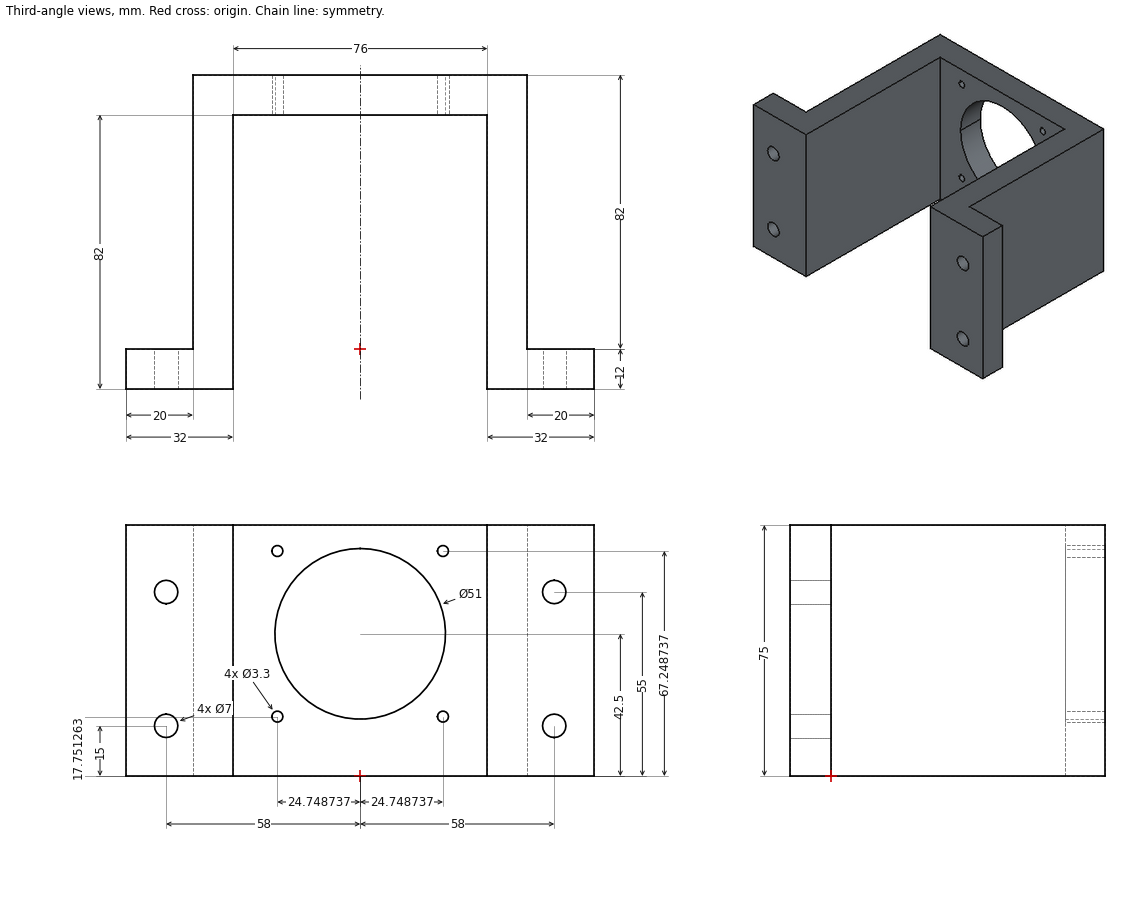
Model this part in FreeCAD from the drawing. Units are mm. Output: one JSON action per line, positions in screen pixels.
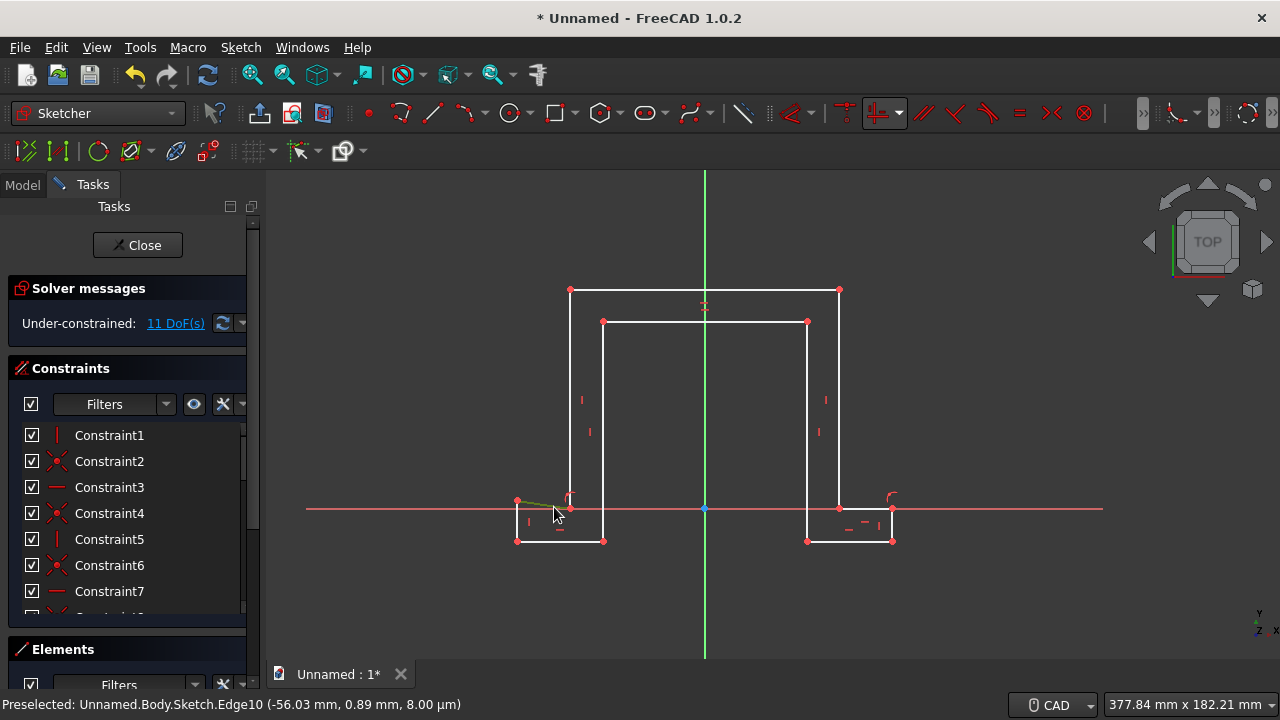
{"action": "key", "text": "h"}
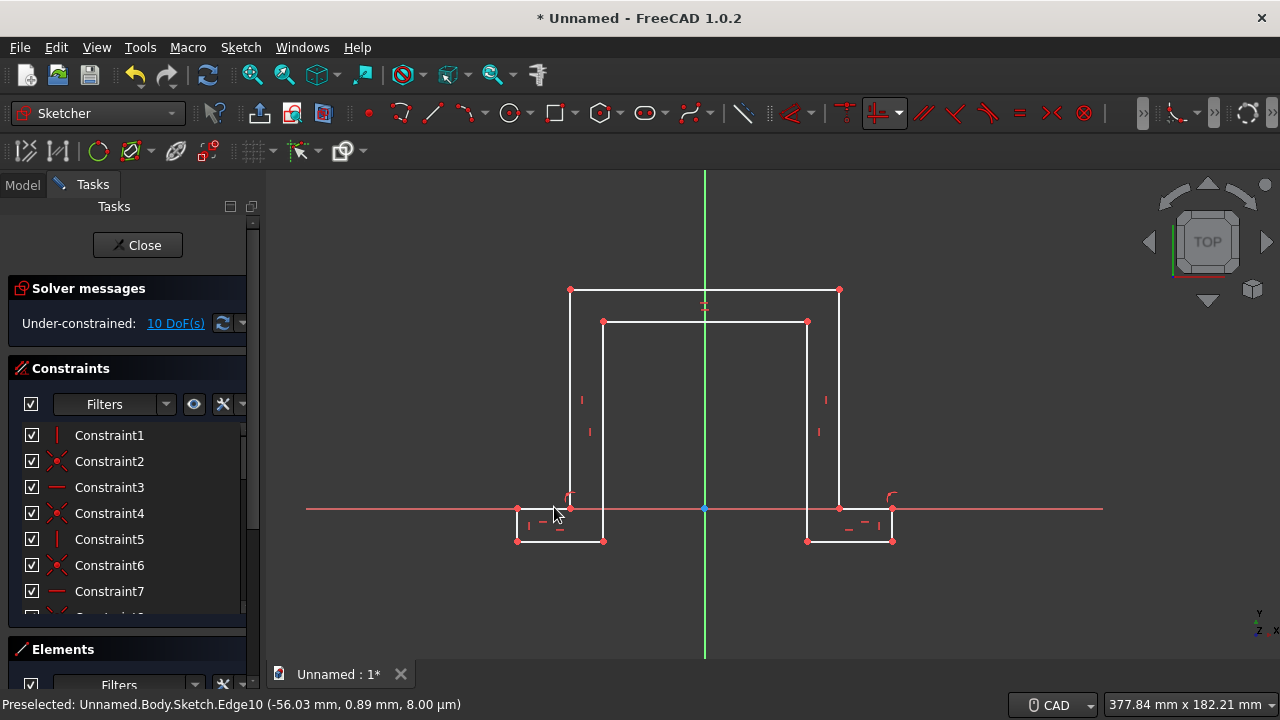
{"action": "left_click", "coordinate": [603, 542]}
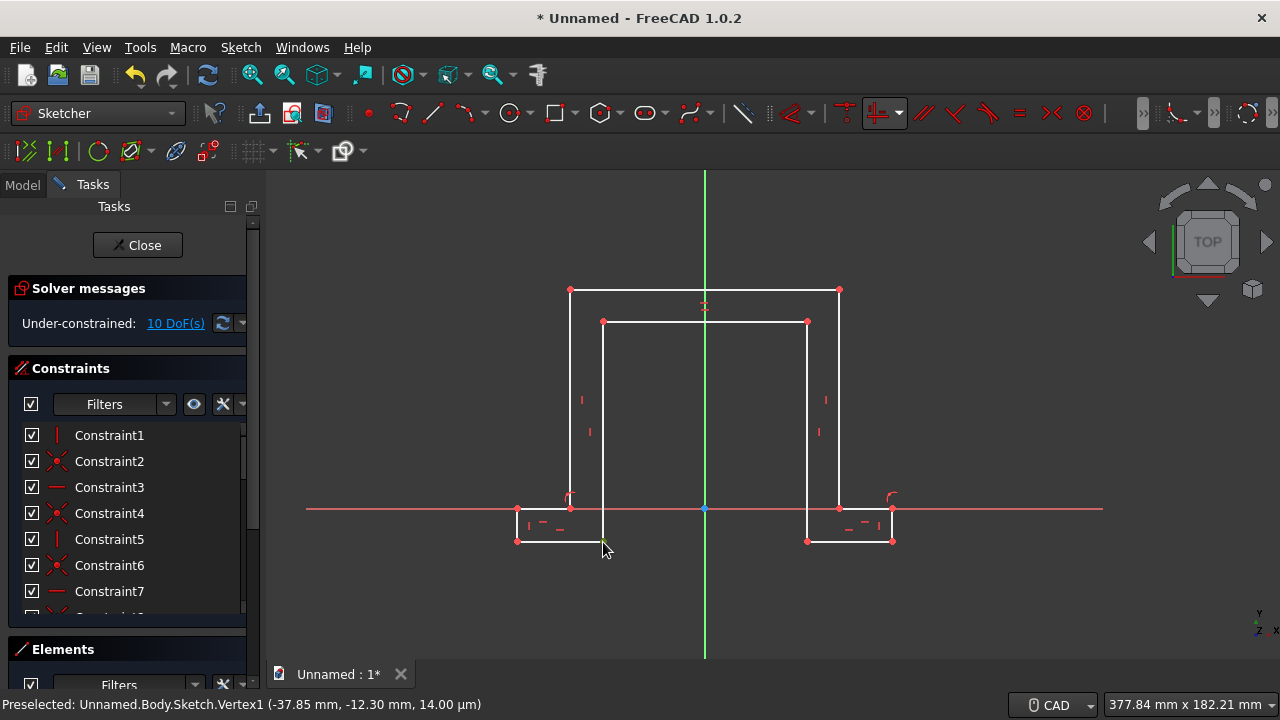
{"action": "left_click", "coordinate": [807, 542]}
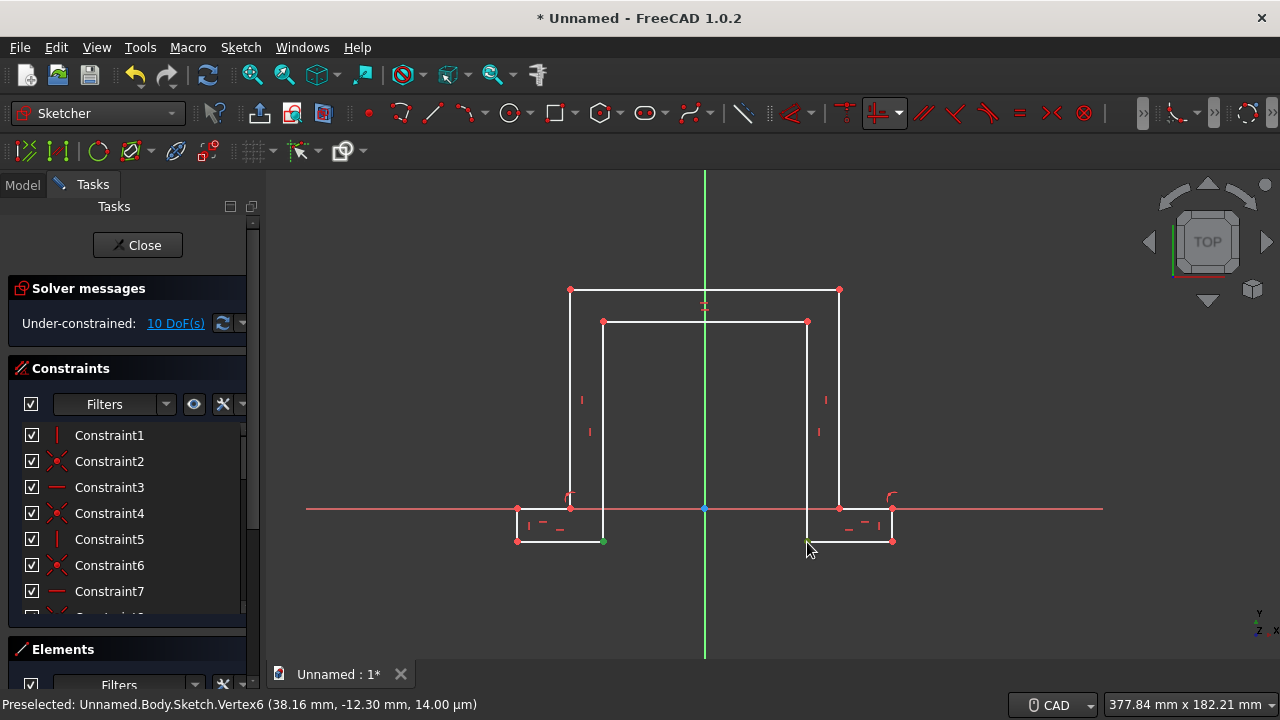
{"action": "left_click", "coordinate": [705, 600]}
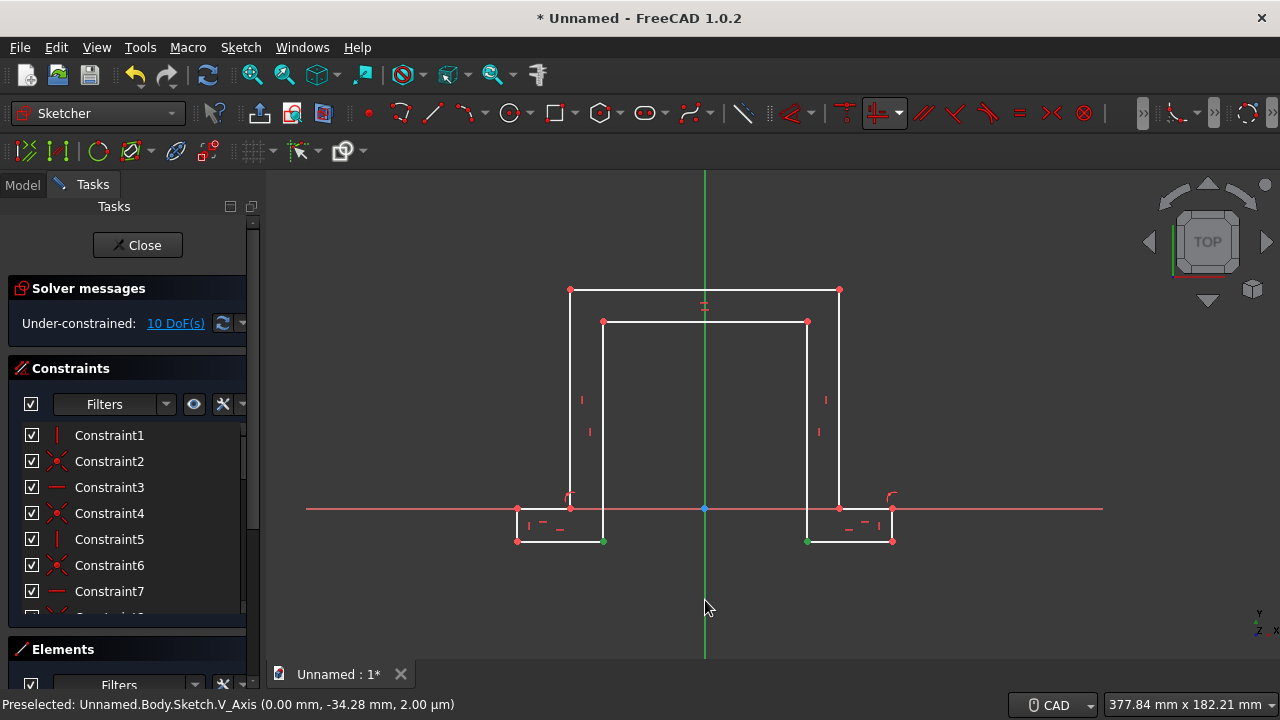
{"action": "left_click", "coordinate": [1052, 114]}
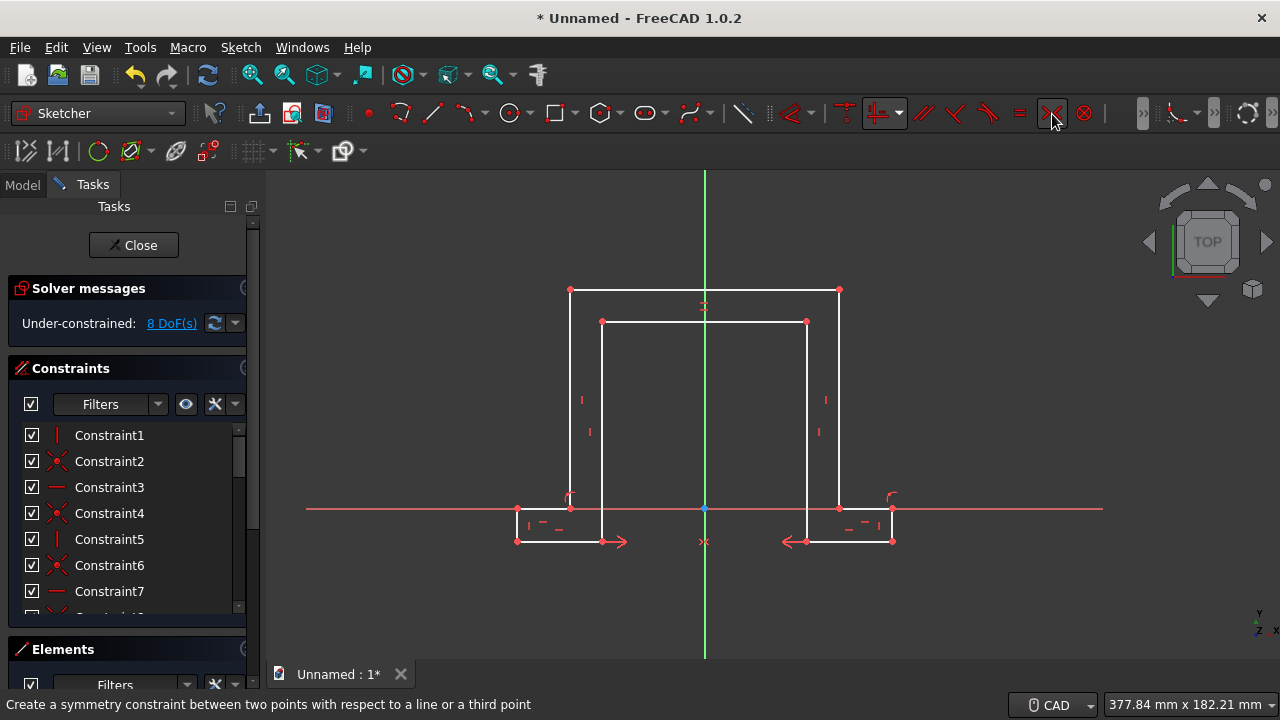
{"action": "left_click", "coordinate": [790, 114]}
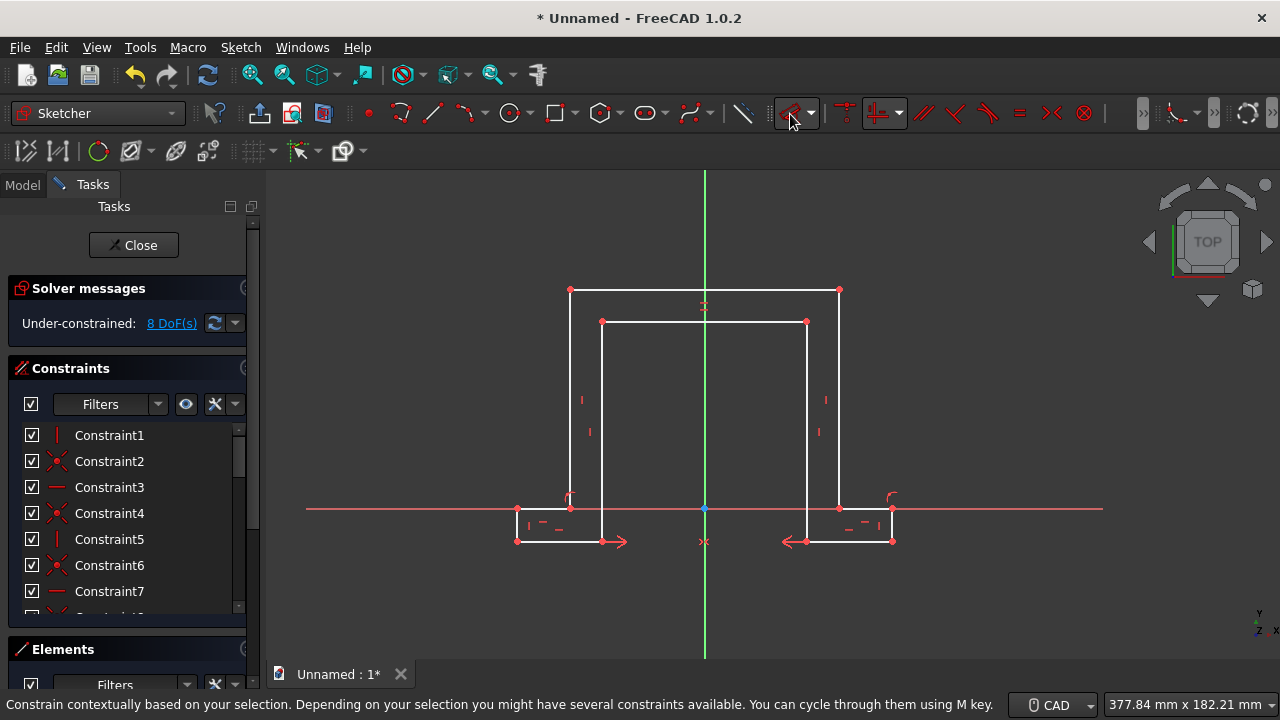
{"action": "left_click", "coordinate": [602, 476]}
{"action": "left_click", "coordinate": [636, 432]}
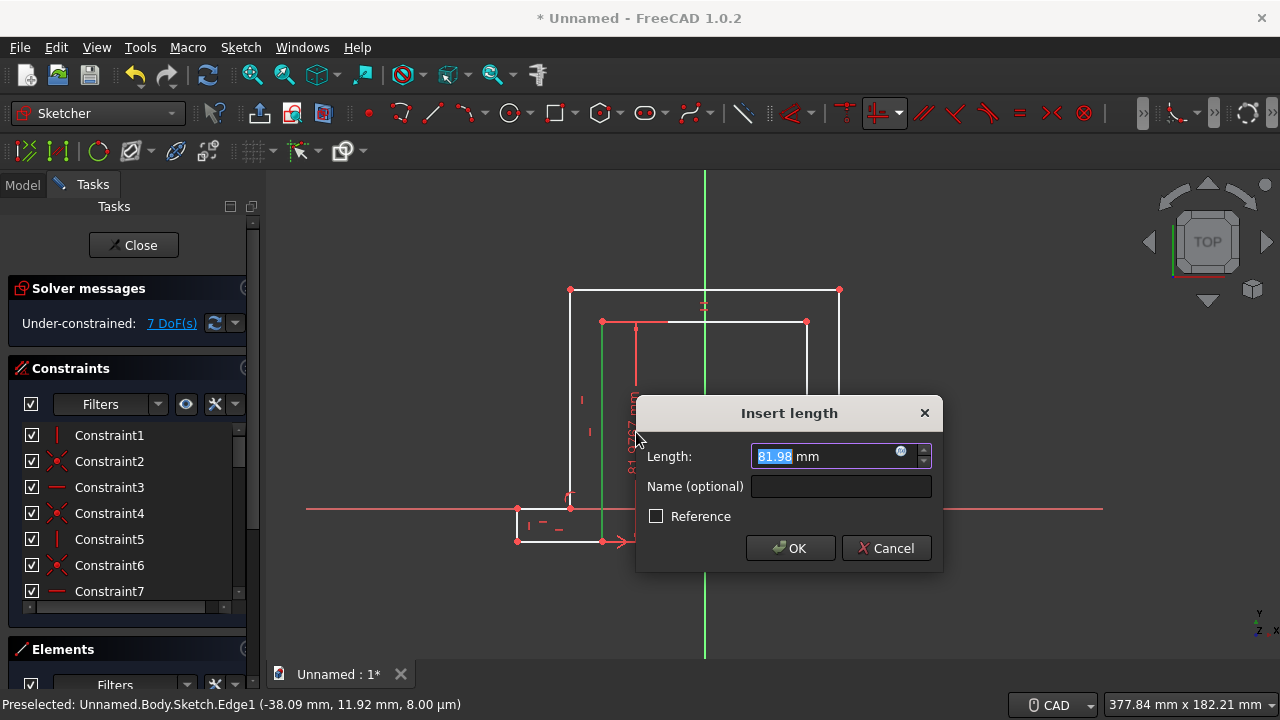
{"action": "type", "text": "82"}
{"action": "key", "text": "Return"}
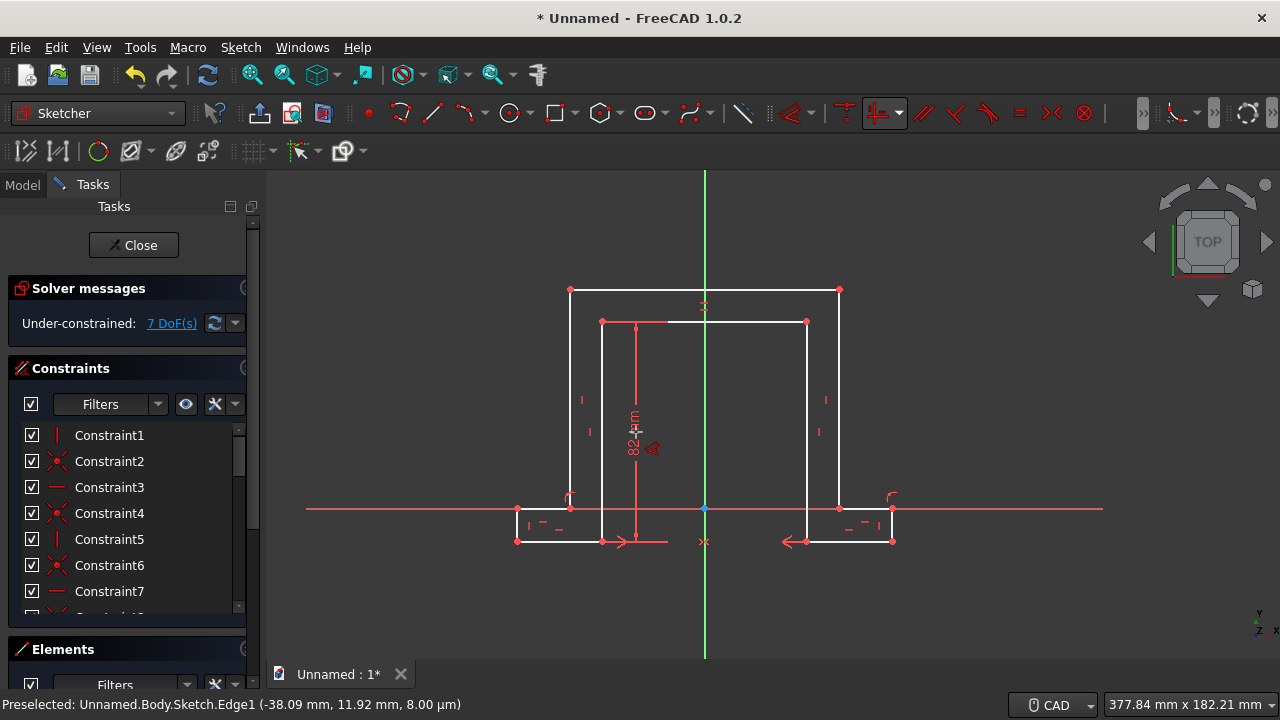
{"action": "left_click", "coordinate": [664, 322]}
{"action": "left_click", "coordinate": [658, 356]}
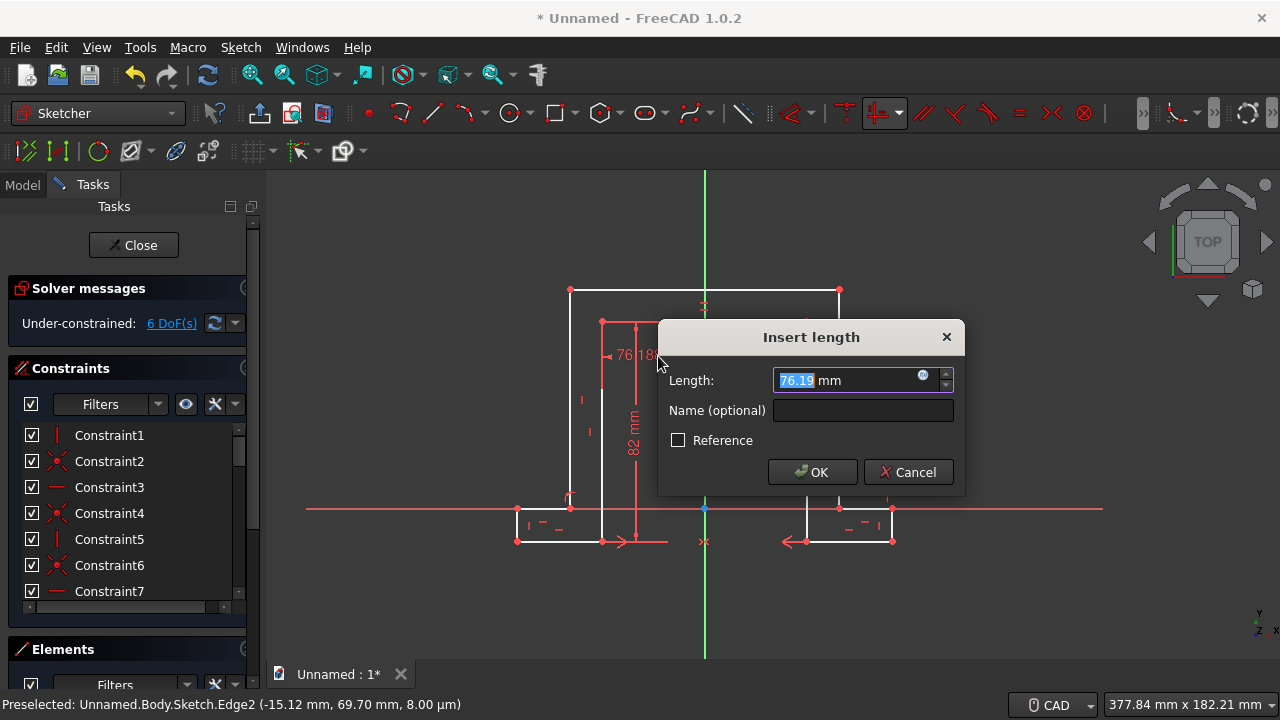
{"action": "type", "text": "76"}
{"action": "key", "text": "Return"}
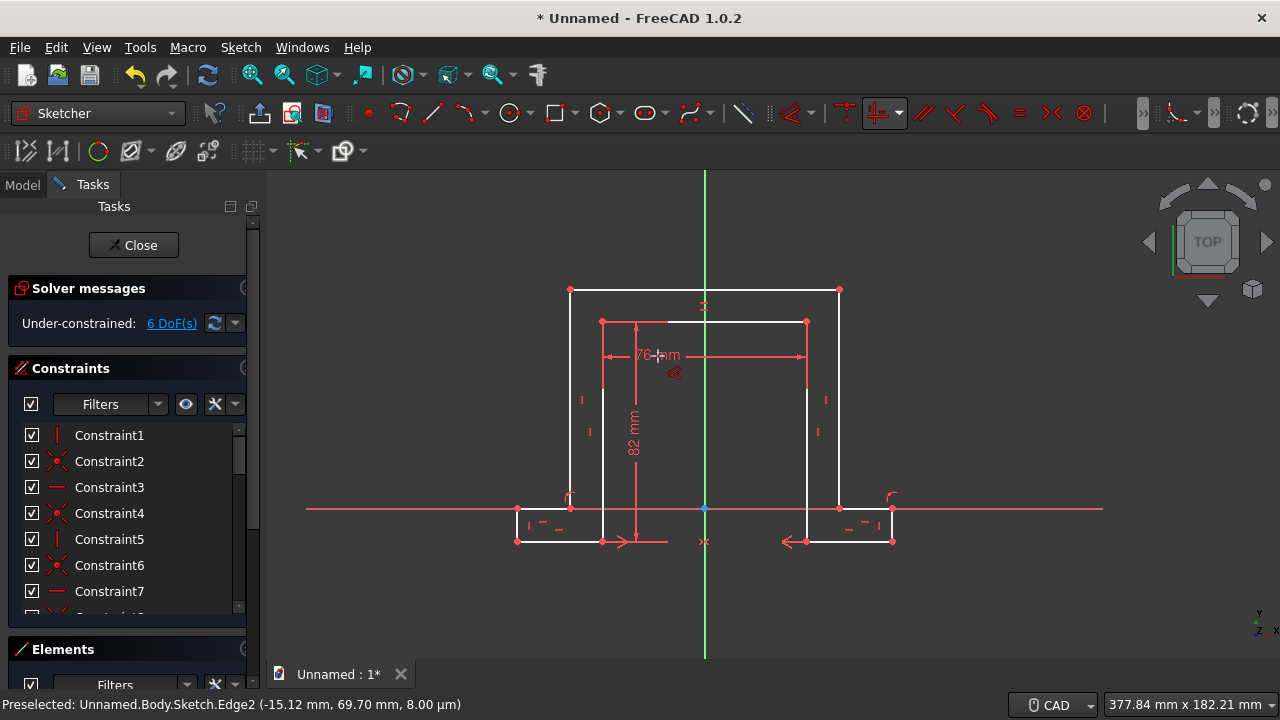
{"action": "left_click", "coordinate": [832, 542]}
{"action": "left_click", "coordinate": [849, 576]}